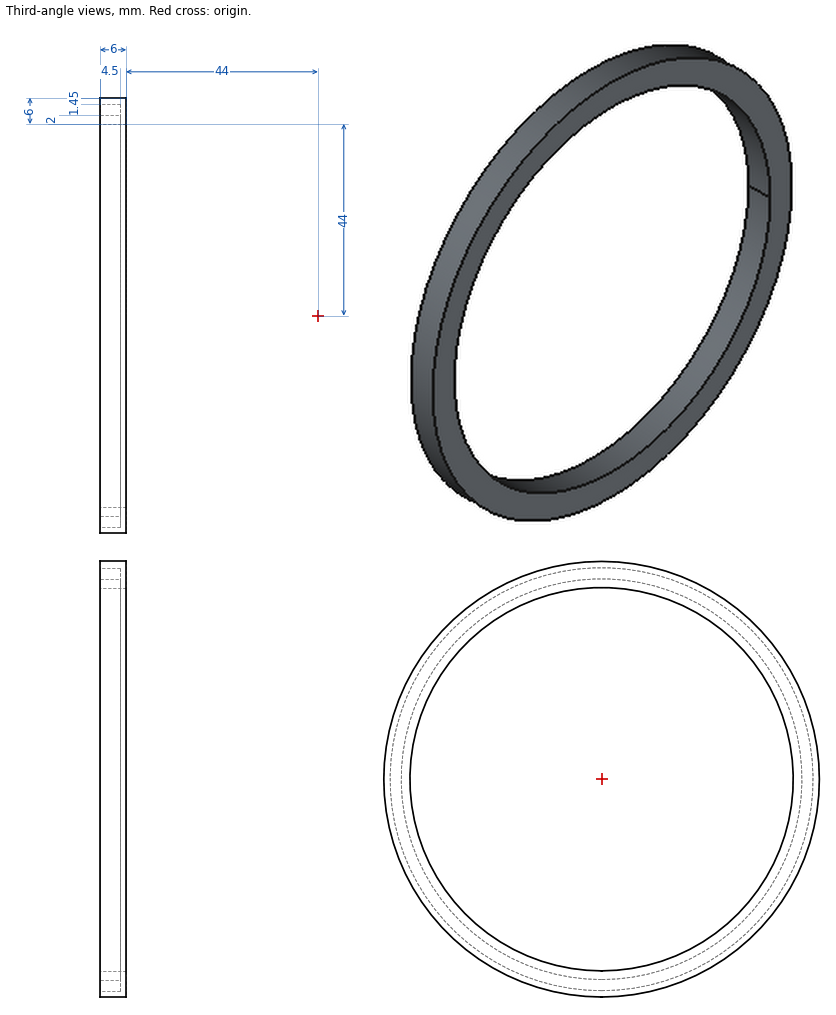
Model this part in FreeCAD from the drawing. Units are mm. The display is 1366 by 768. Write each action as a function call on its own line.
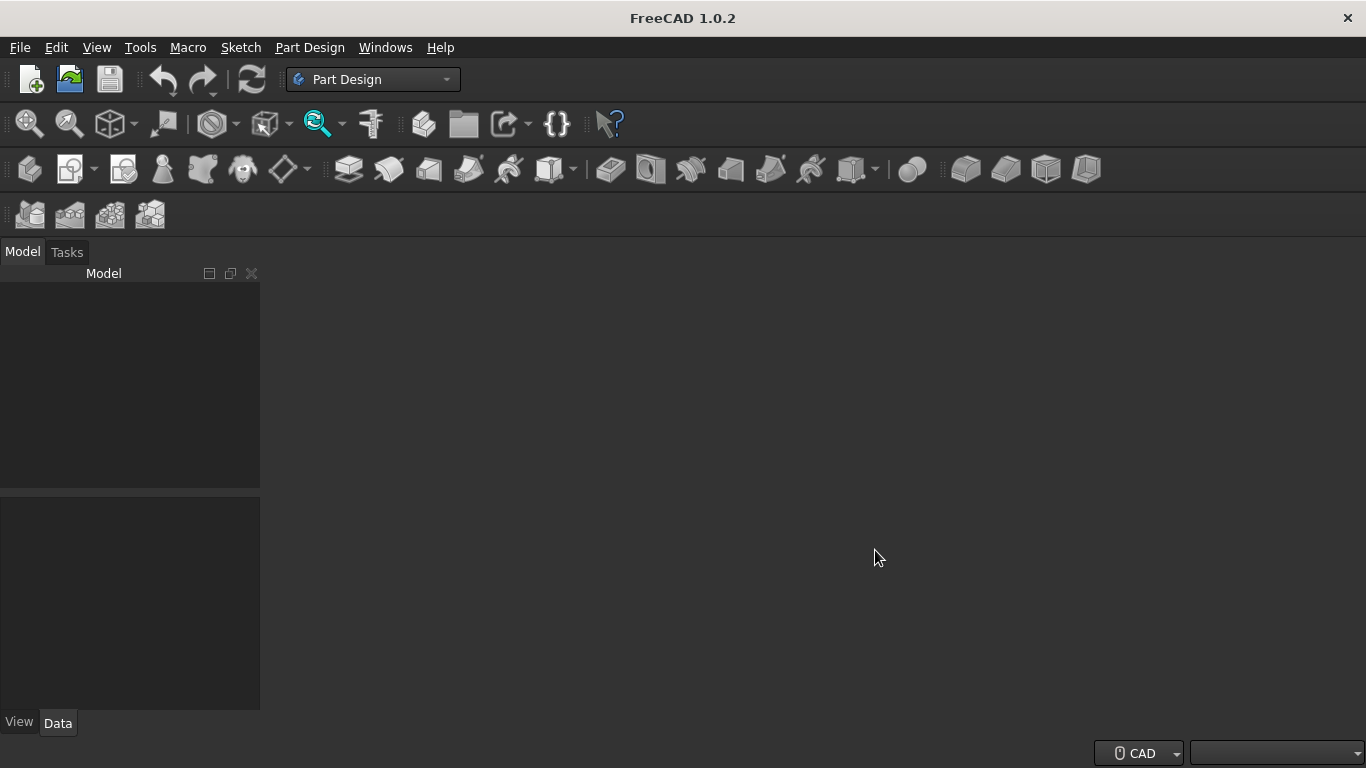
click(30, 80)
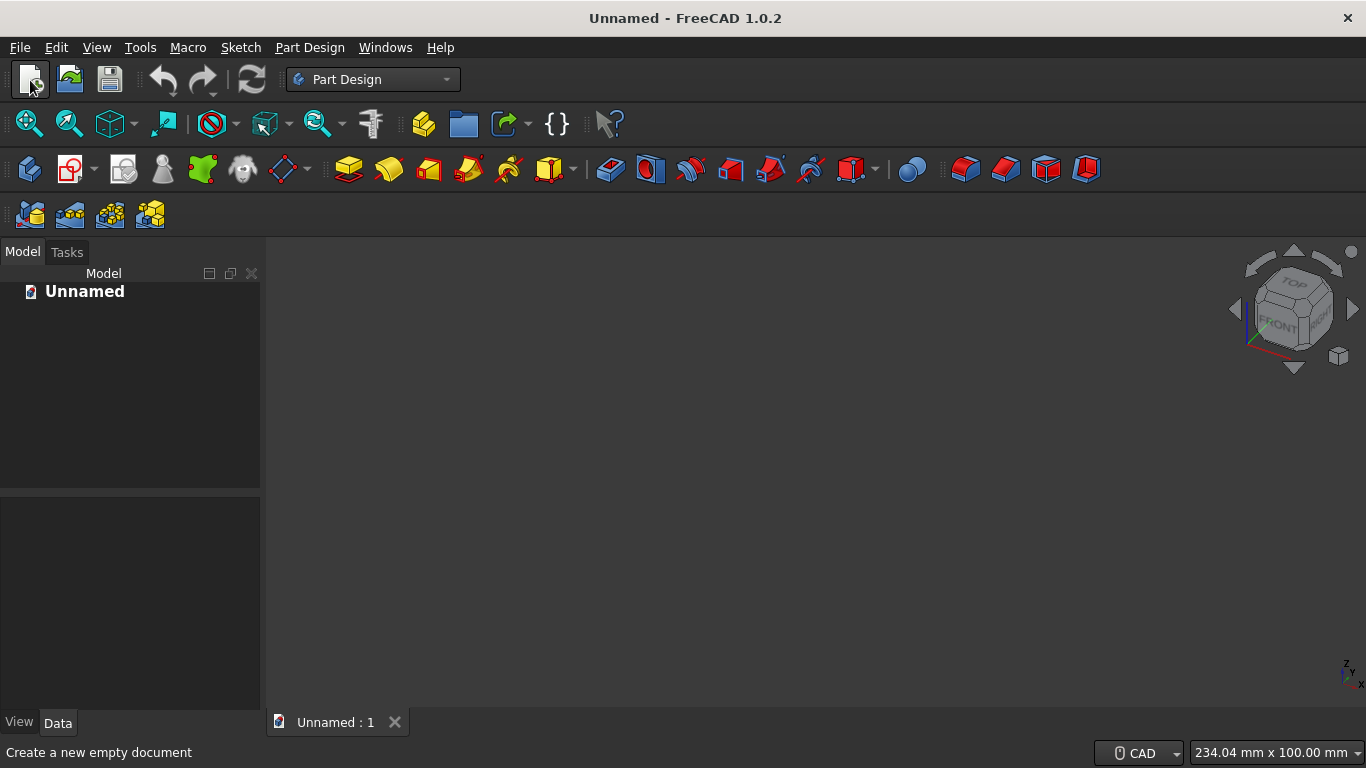
click(70, 170)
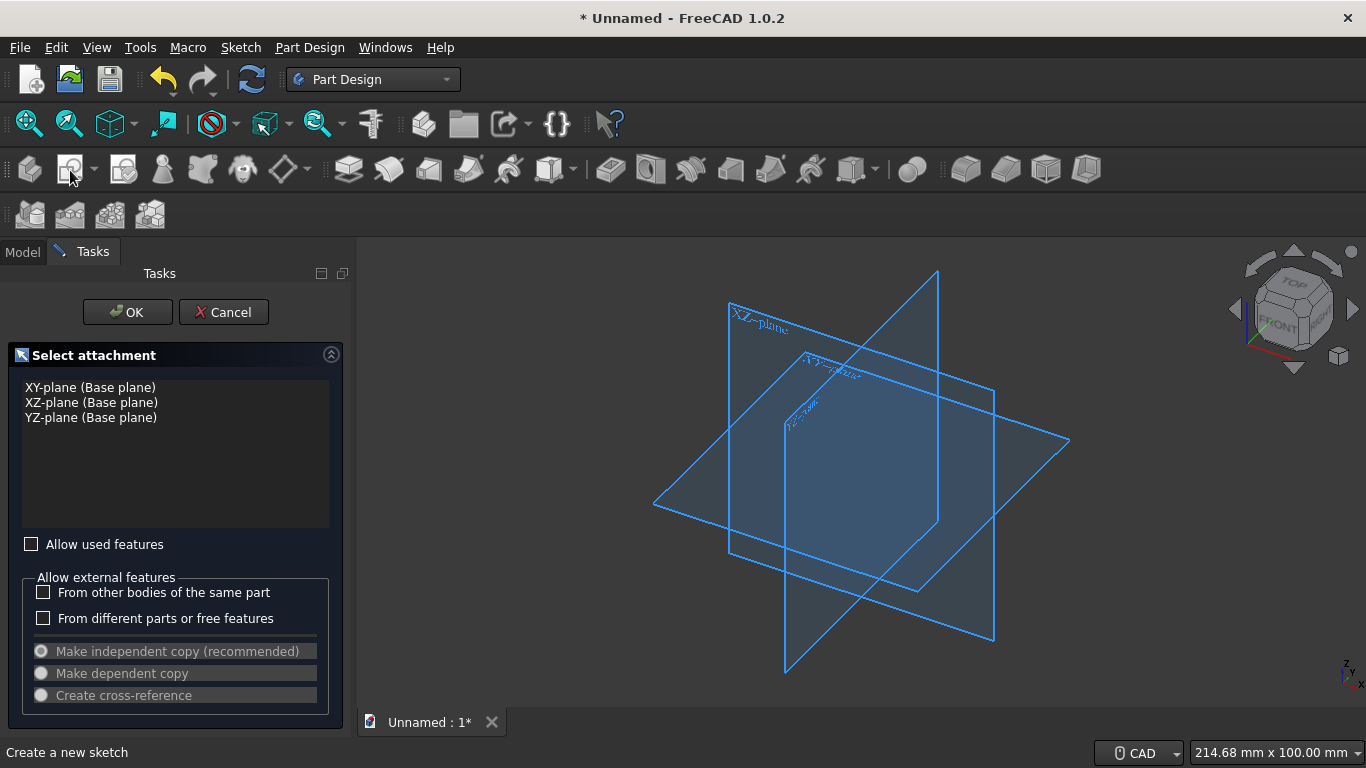
click(82, 388)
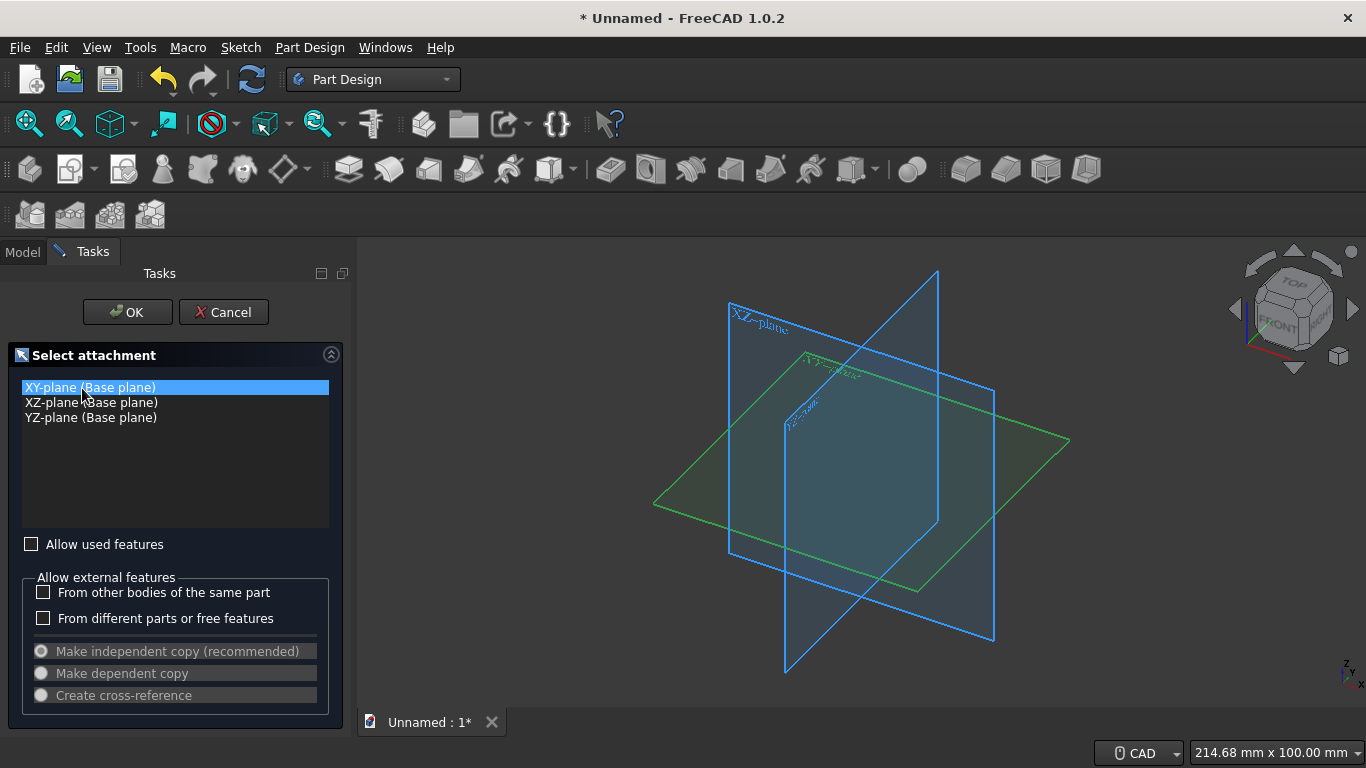
click(128, 312)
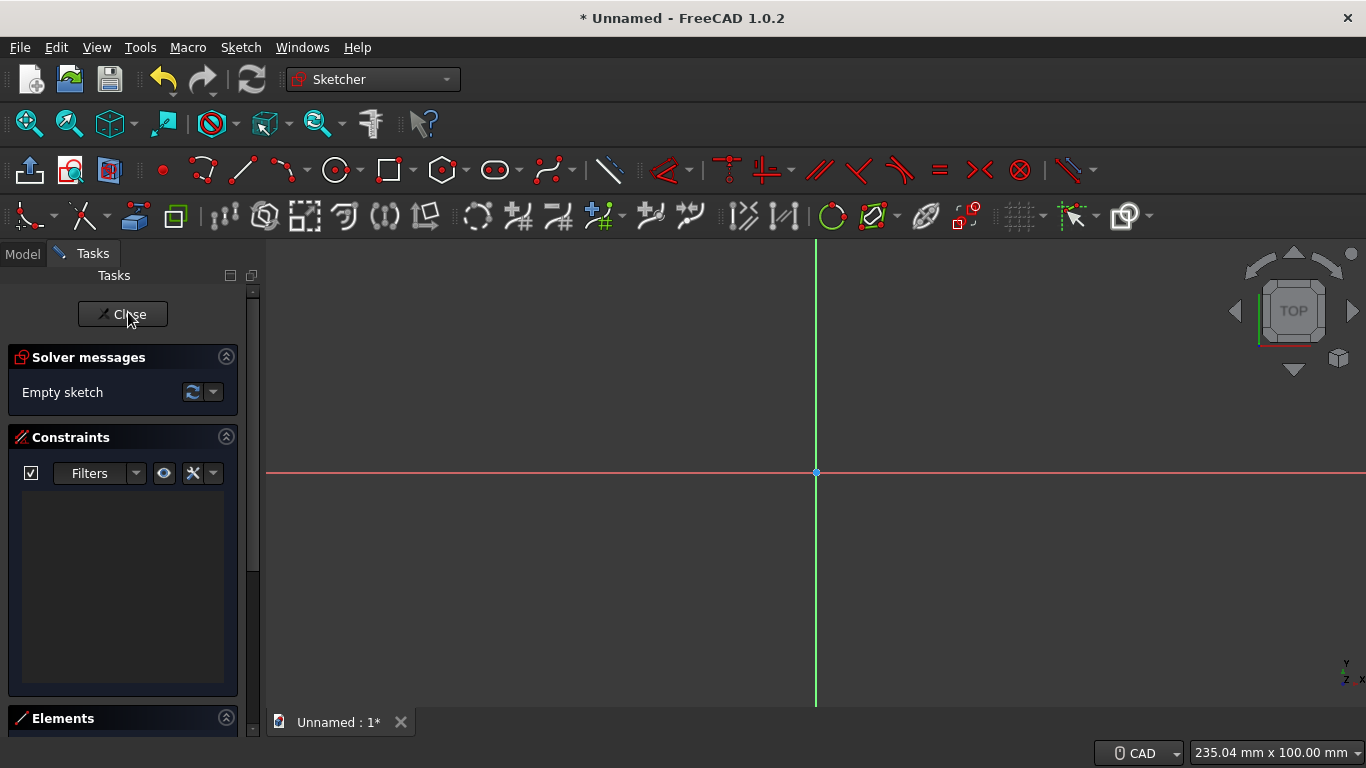
scroll(748, 473, down, 5)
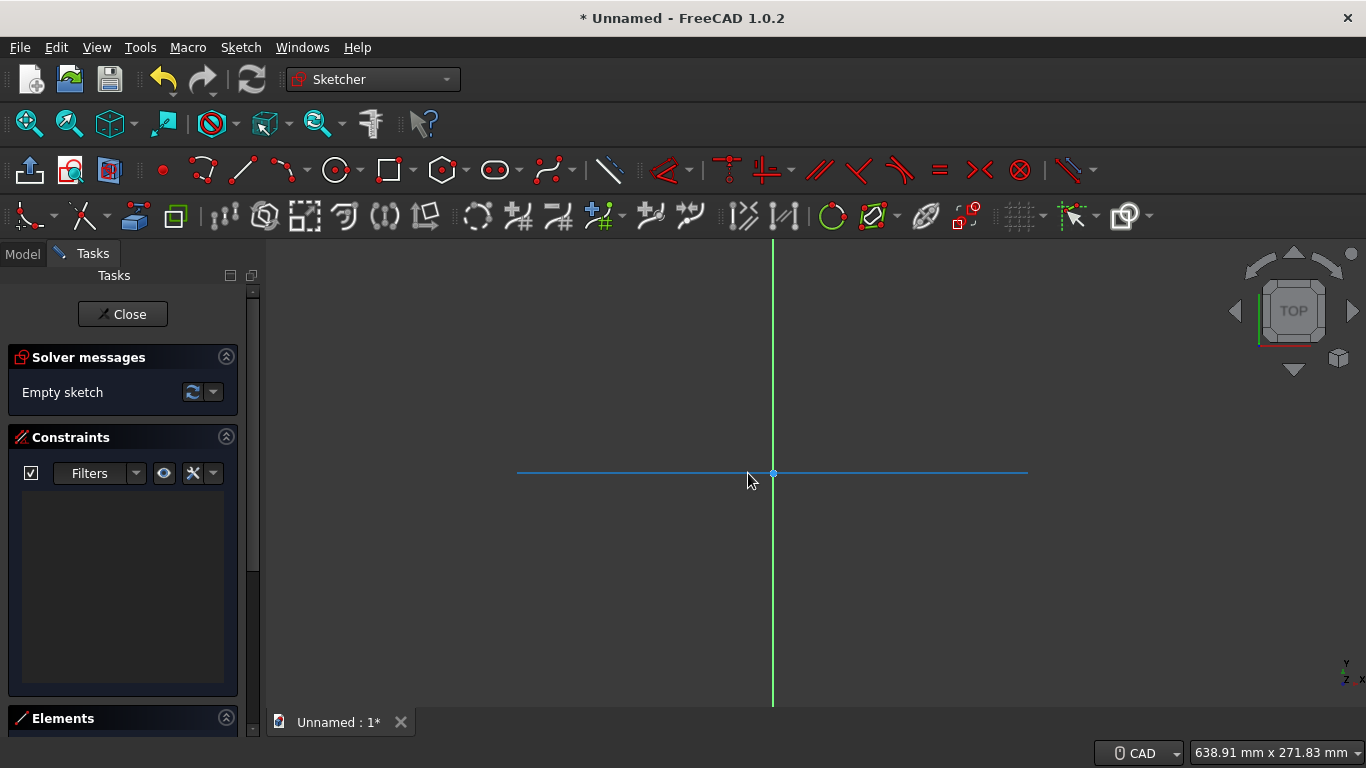
scroll(689, 388, up, 15)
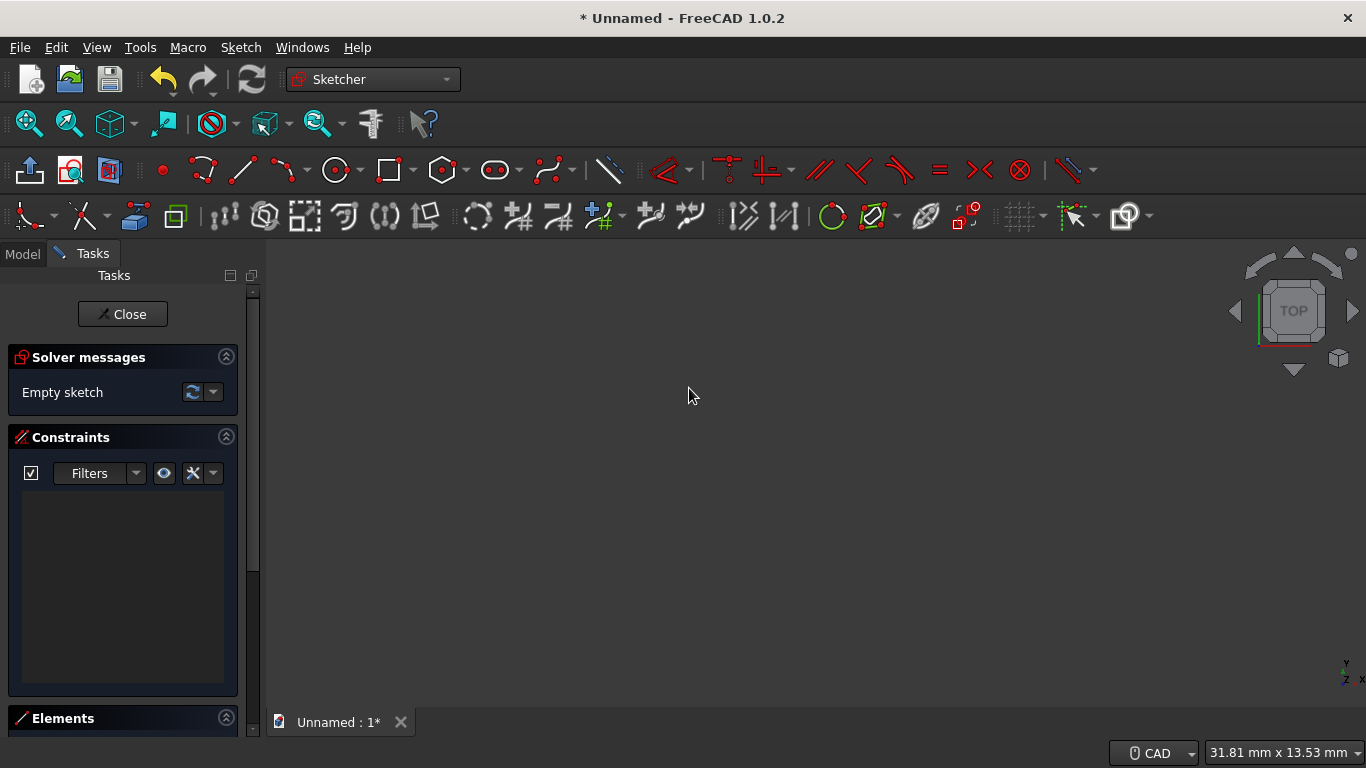
scroll(753, 465, up, 2)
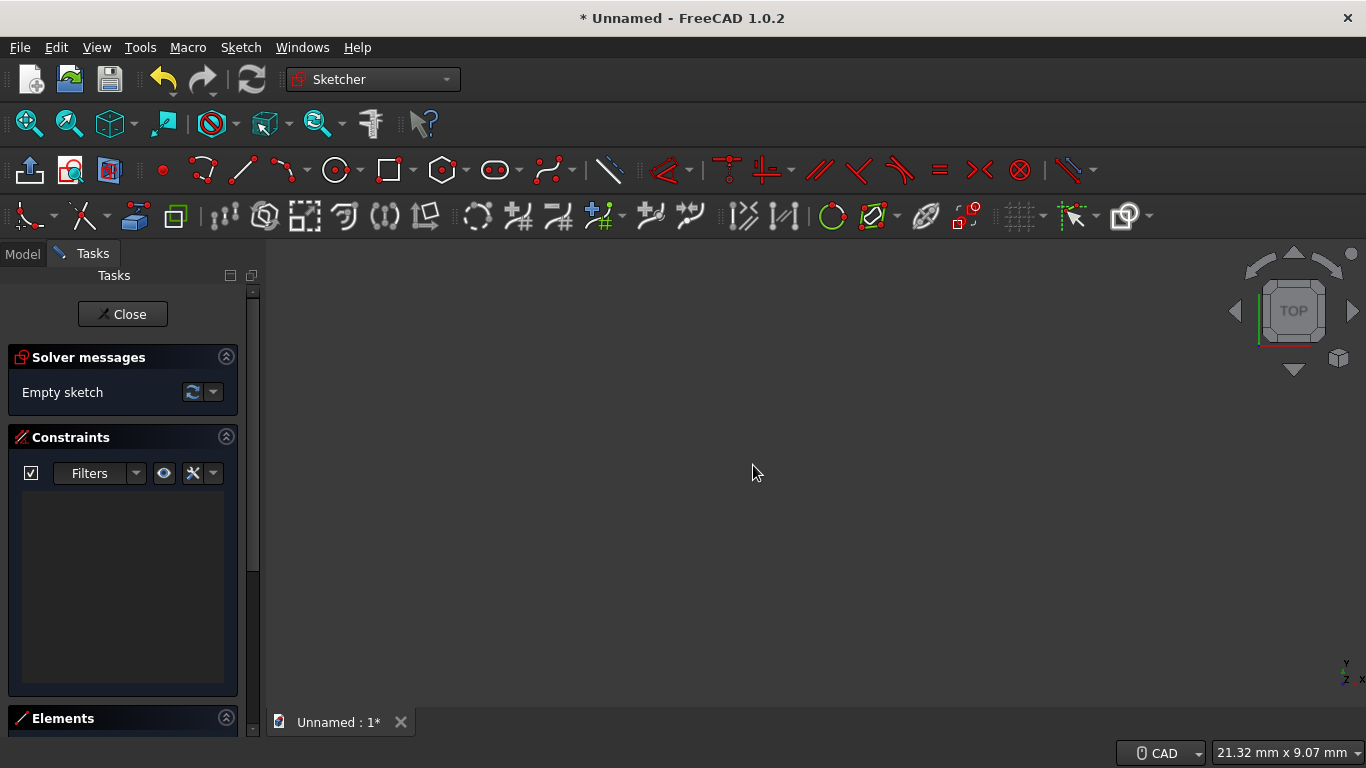
click(204, 170)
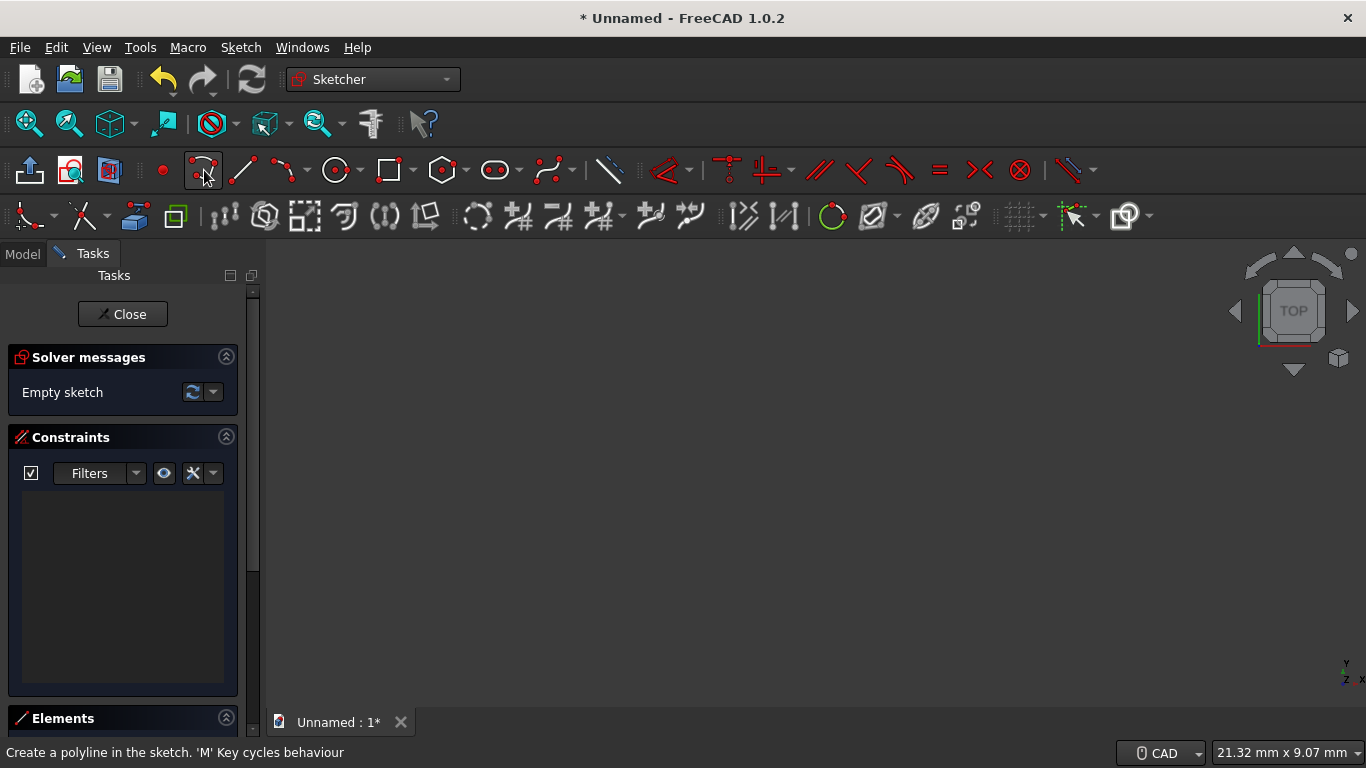
click(902, 627)
click(902, 318)
click(593, 318)
click(593, 393)
click(825, 393)
click(825, 524)
click(593, 524)
click(593, 627)
click(902, 628)
key(Escape)
key(Escape)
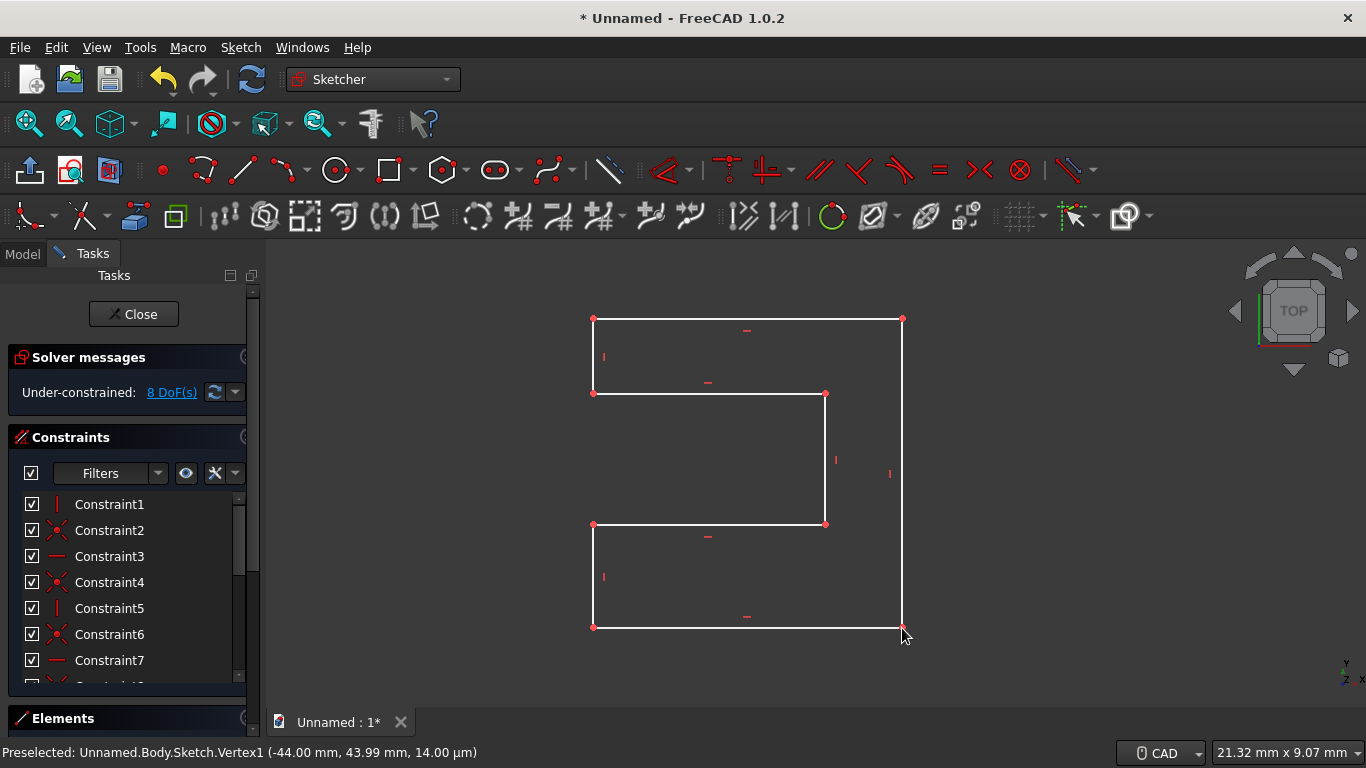
click(664, 170)